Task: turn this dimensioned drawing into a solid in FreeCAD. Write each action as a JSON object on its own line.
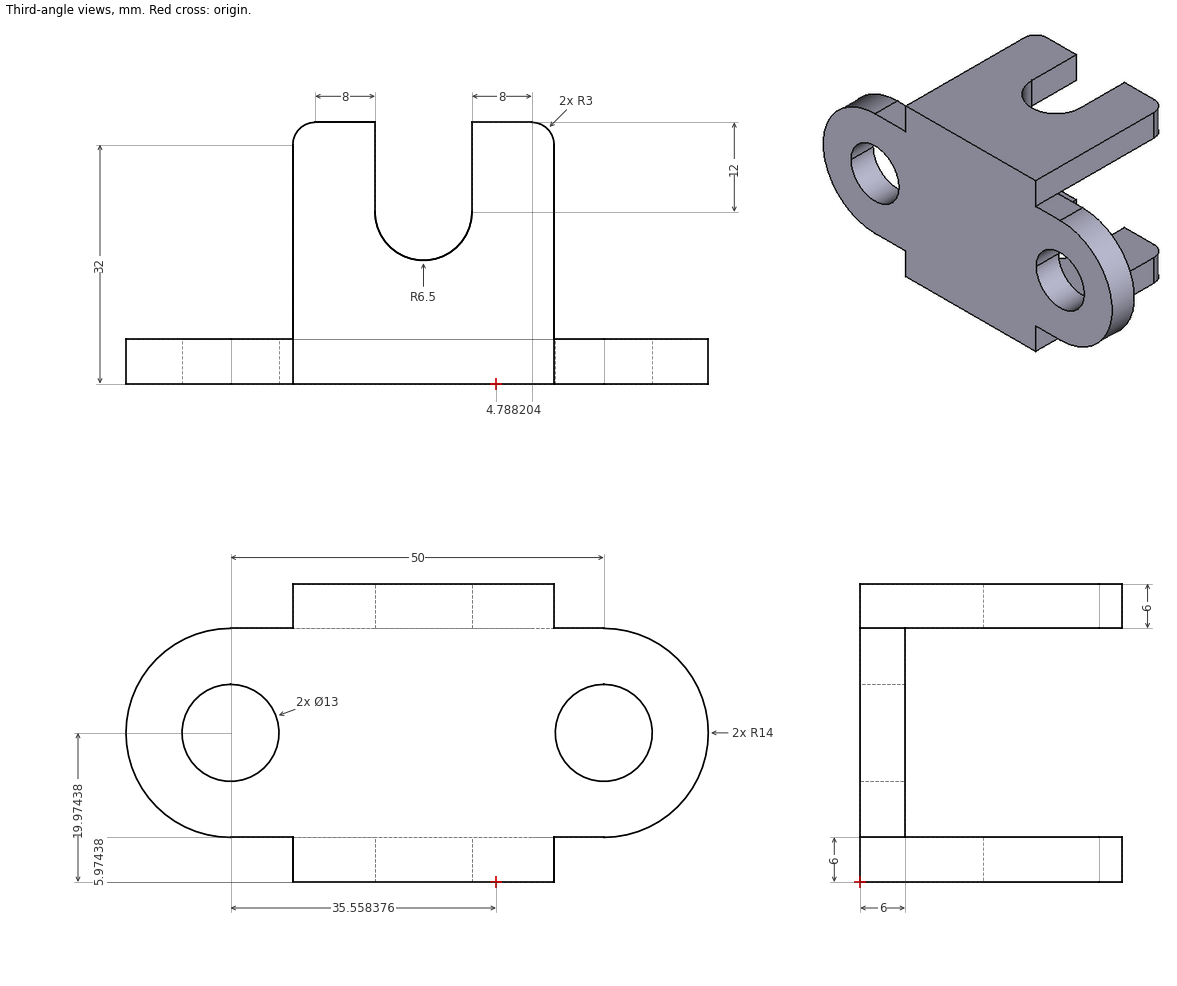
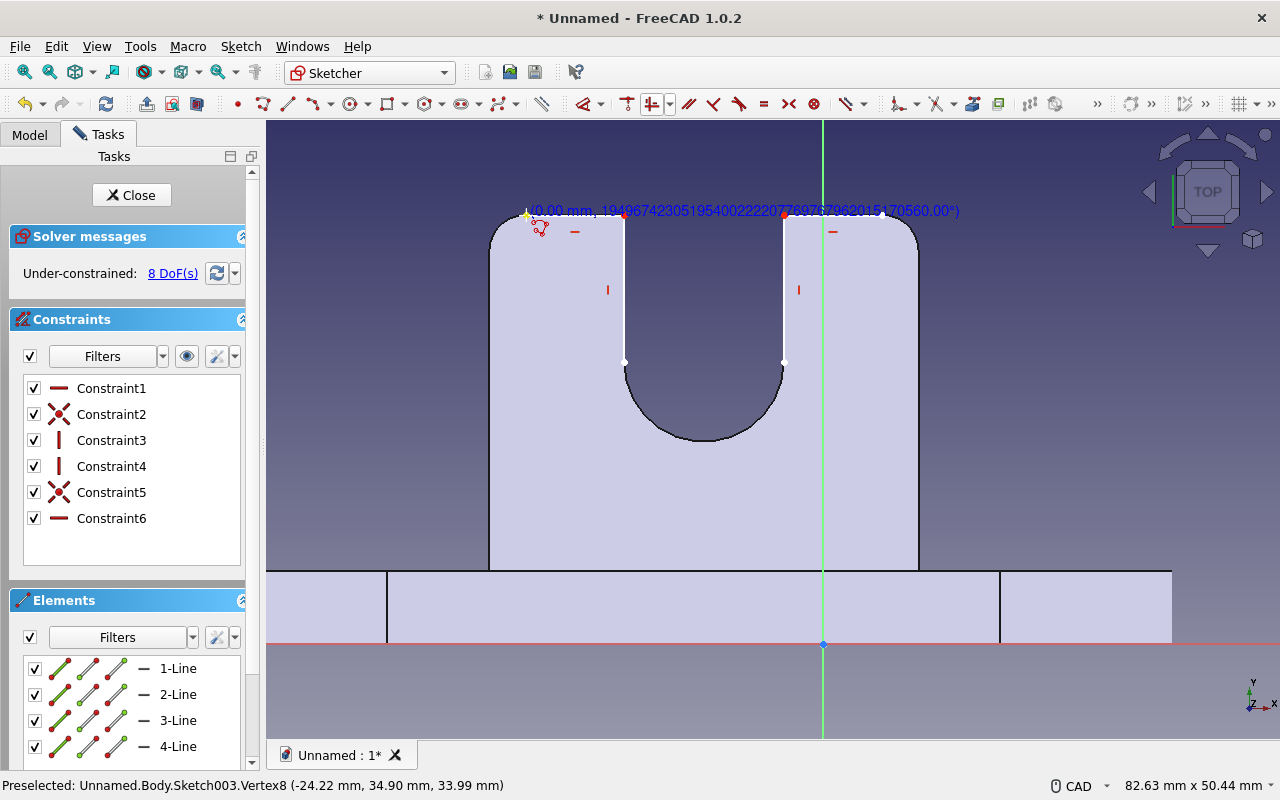
{"action": "left_click", "coordinate": [489, 252]}
{"action": "left_click", "coordinate": [489, 644]}
{"action": "left_click", "coordinate": [919, 635]}
{"action": "left_click", "coordinate": [919, 252]}
{"action": "right_click", "coordinate": [919, 252]}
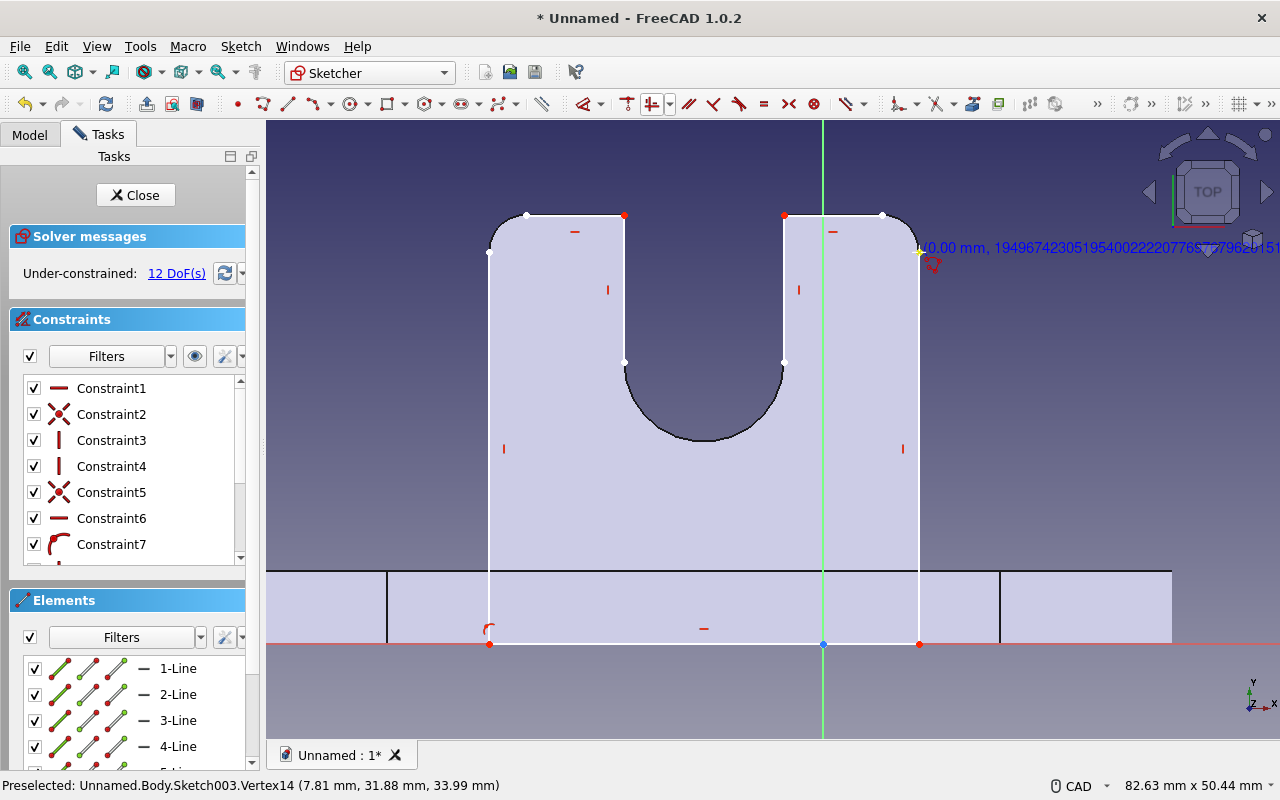
{"action": "left_click", "coordinate": [312, 104]}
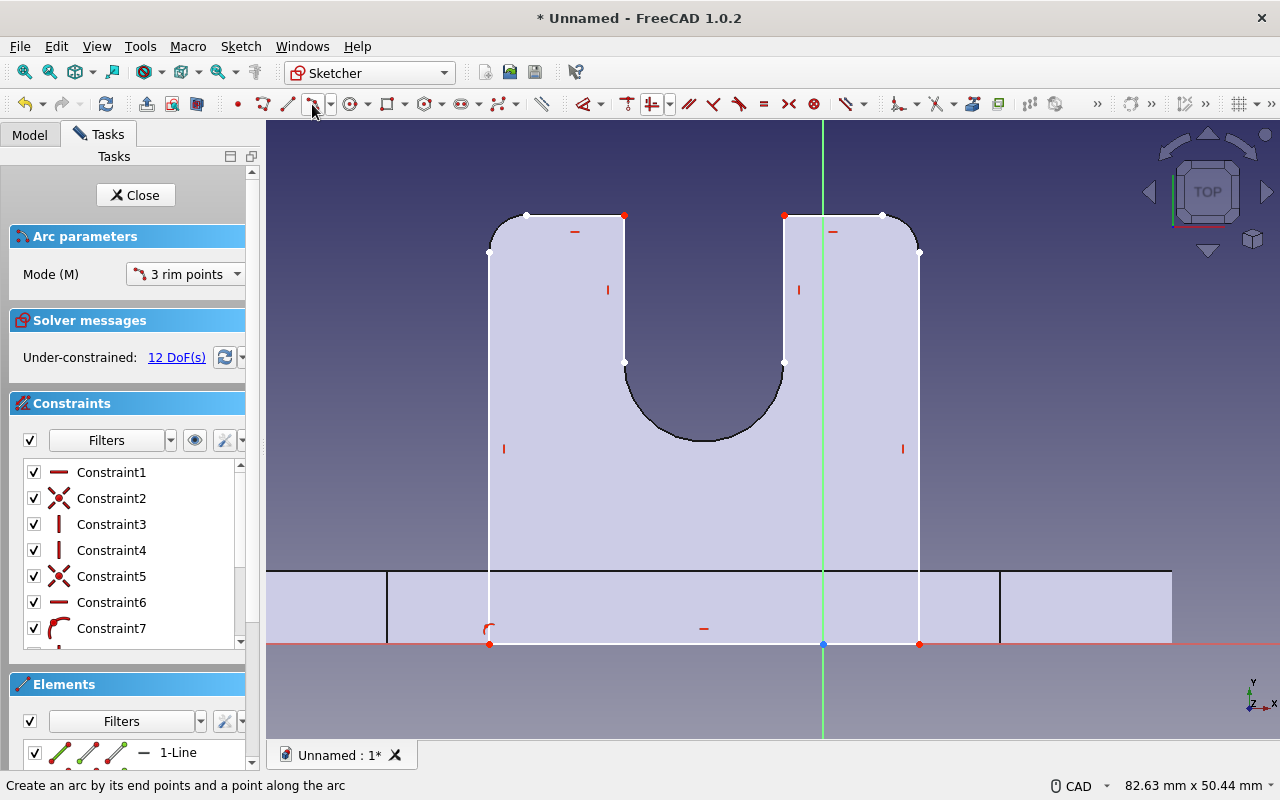
{"action": "left_click", "coordinate": [784, 363]}
{"action": "left_click", "coordinate": [624, 363]}
{"action": "left_click", "coordinate": [704, 442]}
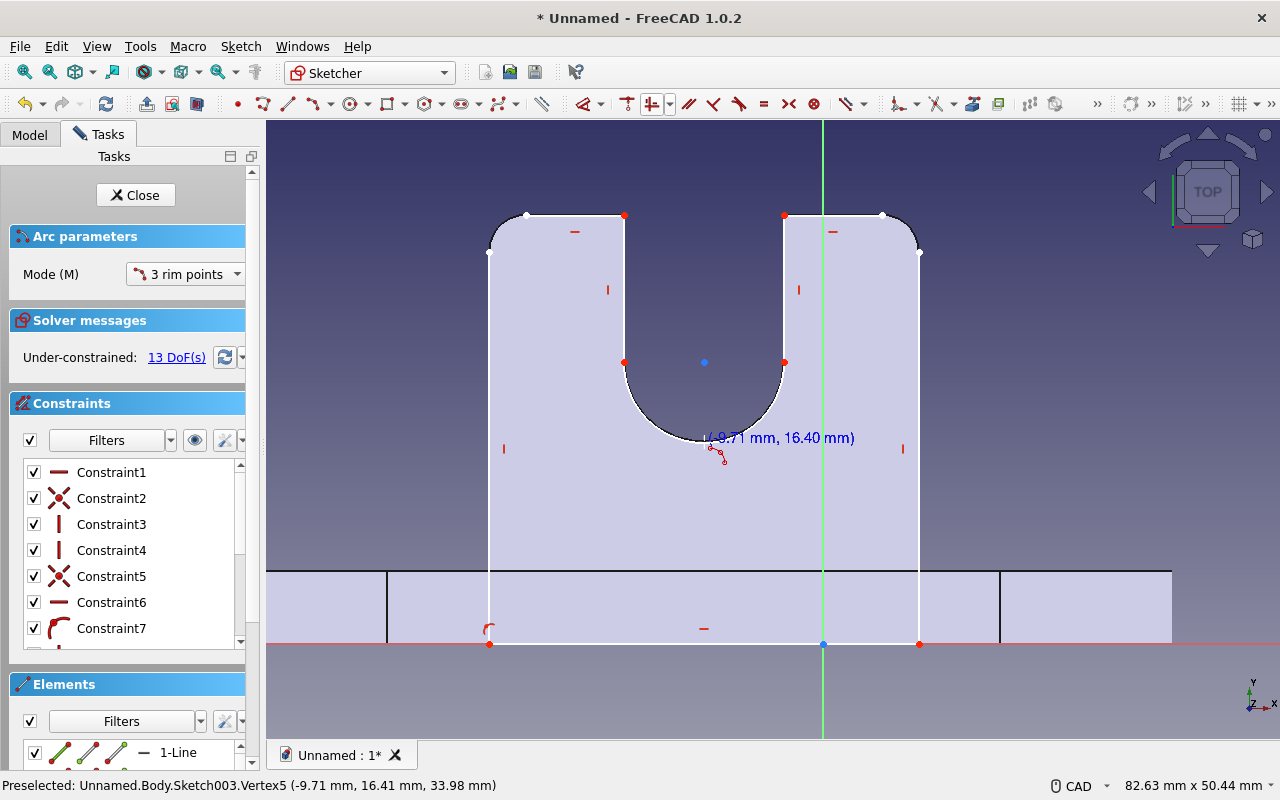
{"action": "left_click", "coordinate": [526, 216]}
{"action": "left_click", "coordinate": [489, 253]}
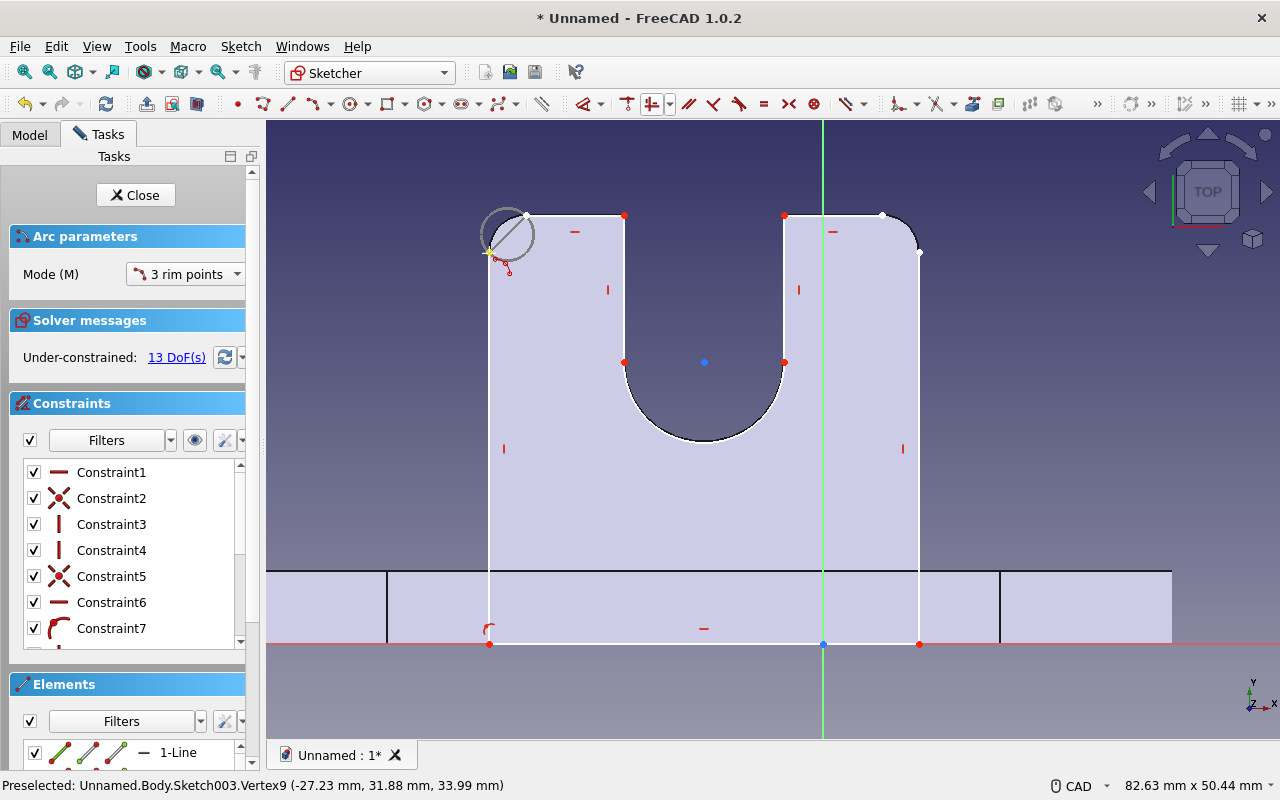
{"action": "scroll", "coordinate": [500, 226], "scroll_direction": "up", "scroll_amount": 2}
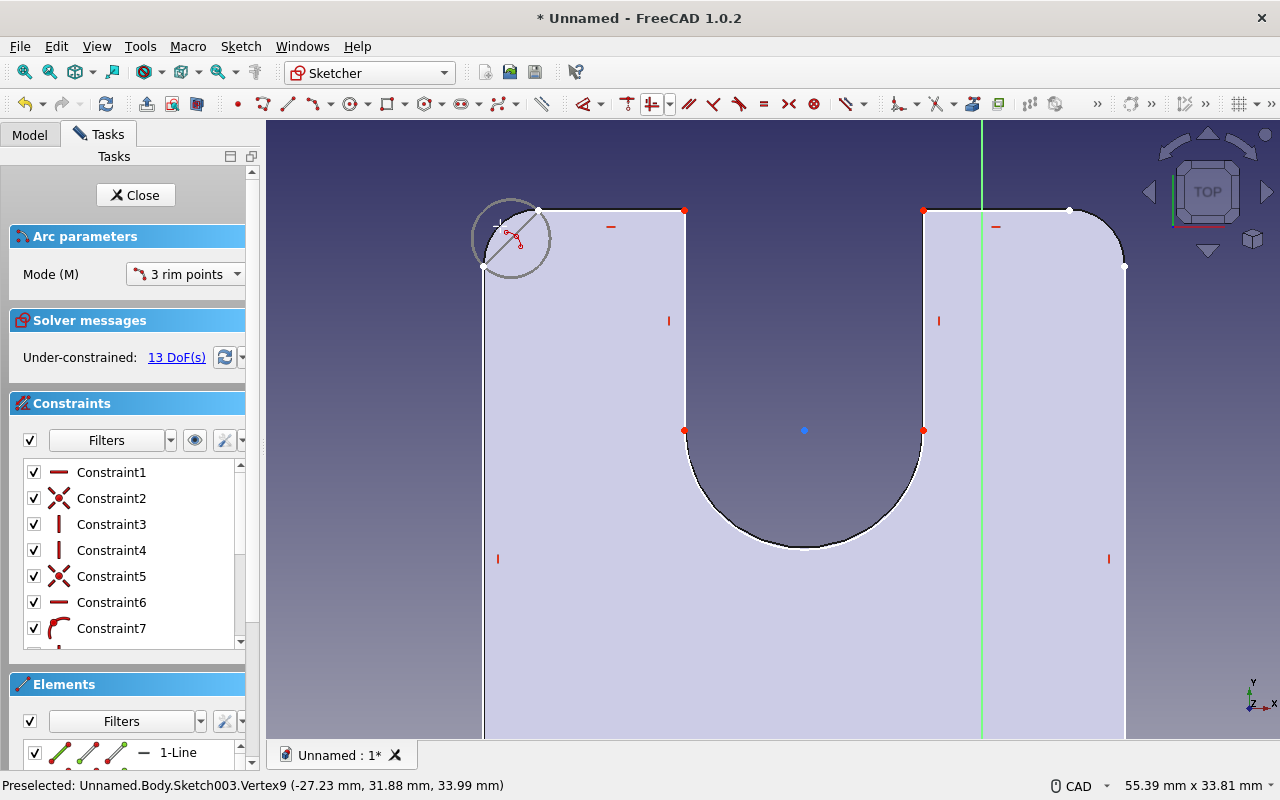
{"action": "left_click", "coordinate": [500, 225]}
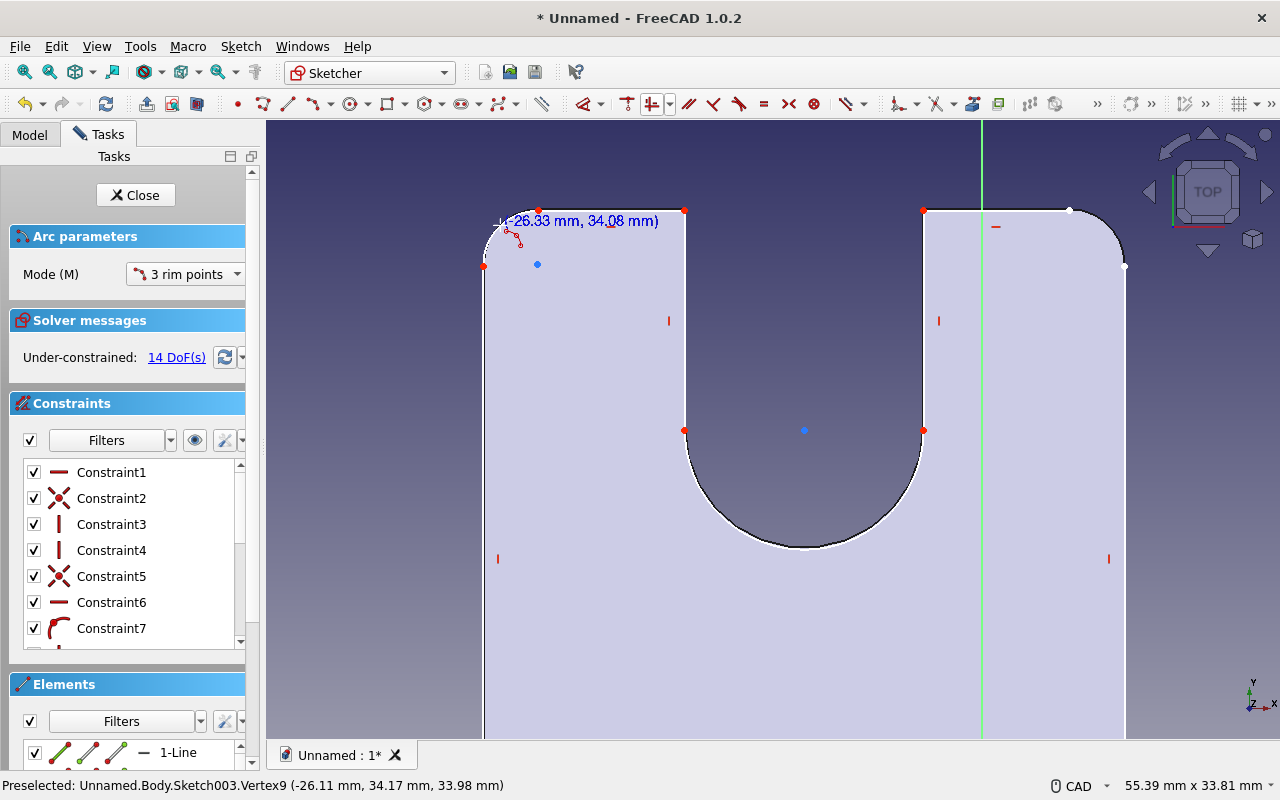
{"action": "scroll", "coordinate": [502, 226], "scroll_direction": "down", "scroll_amount": 2}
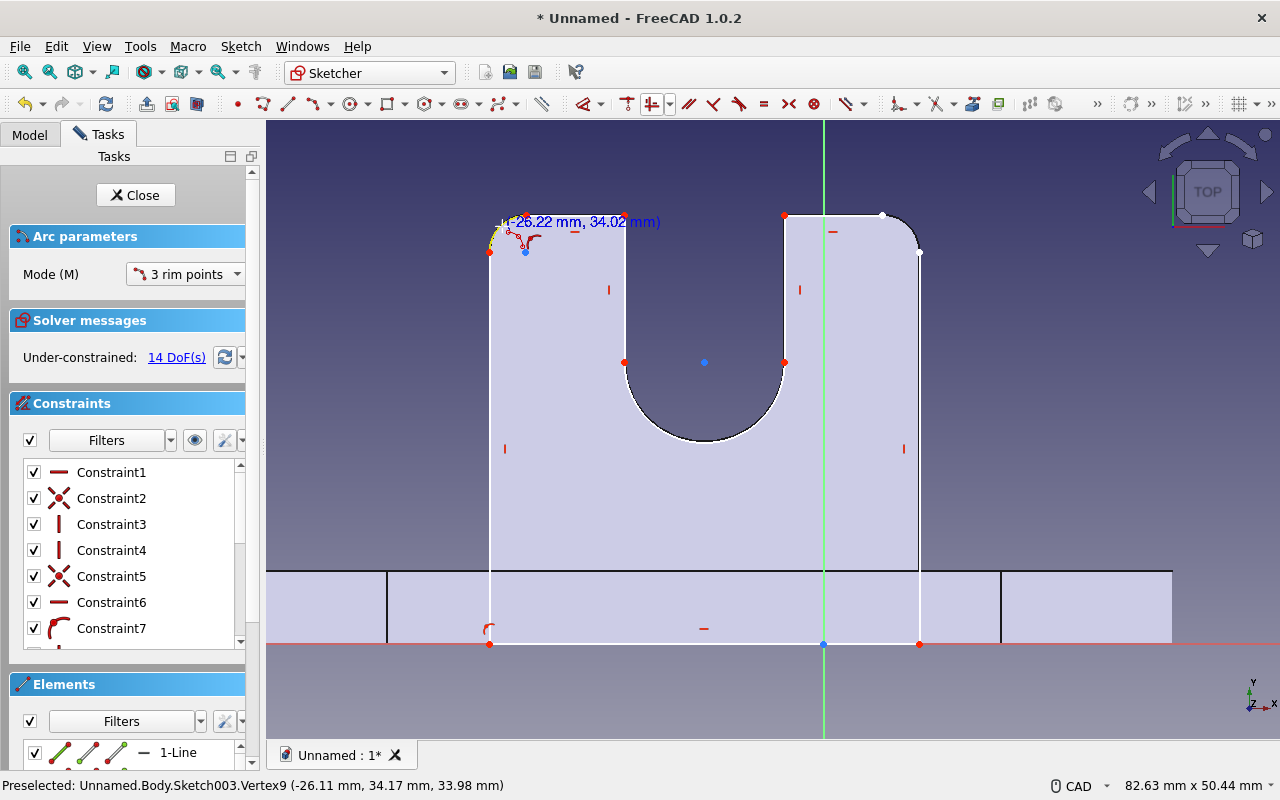
{"action": "left_click", "coordinate": [920, 253]}
{"action": "left_click", "coordinate": [883, 216]}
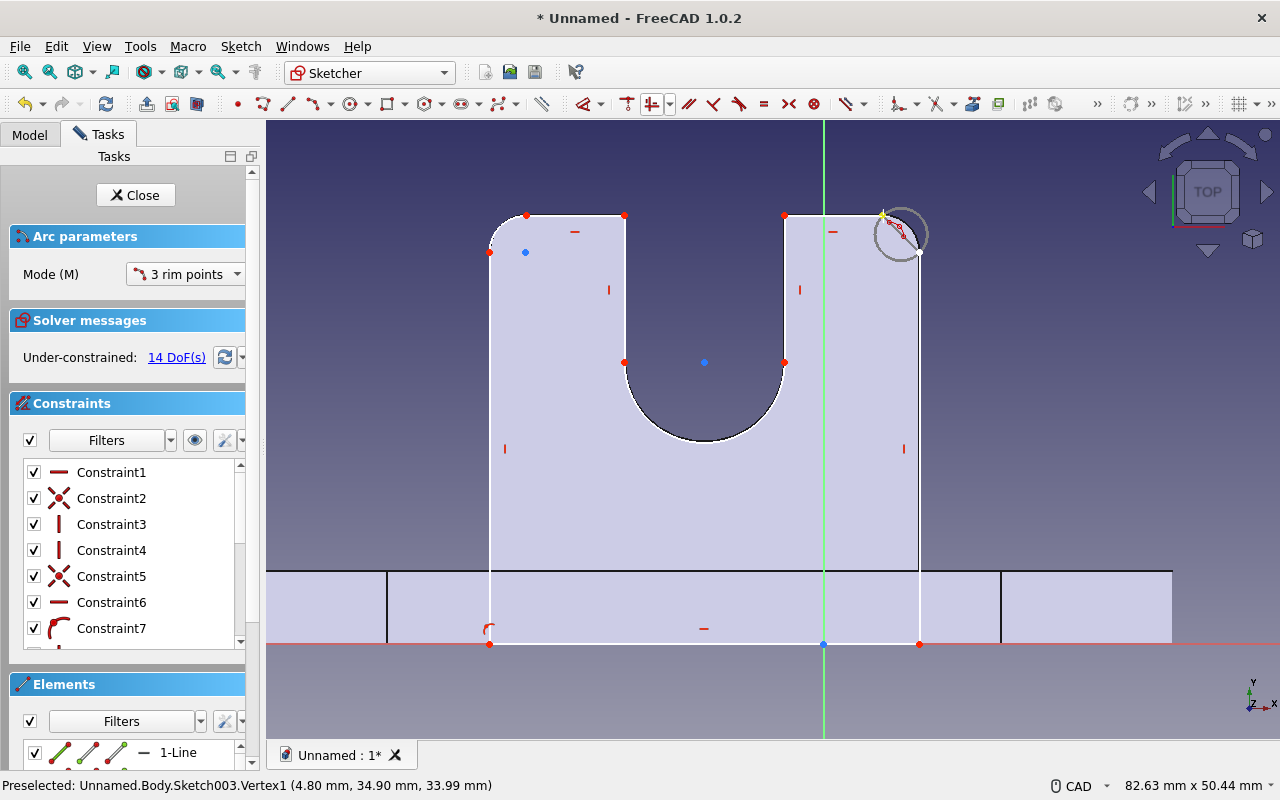
{"action": "scroll", "coordinate": [909, 226], "scroll_direction": "up", "scroll_amount": 2}